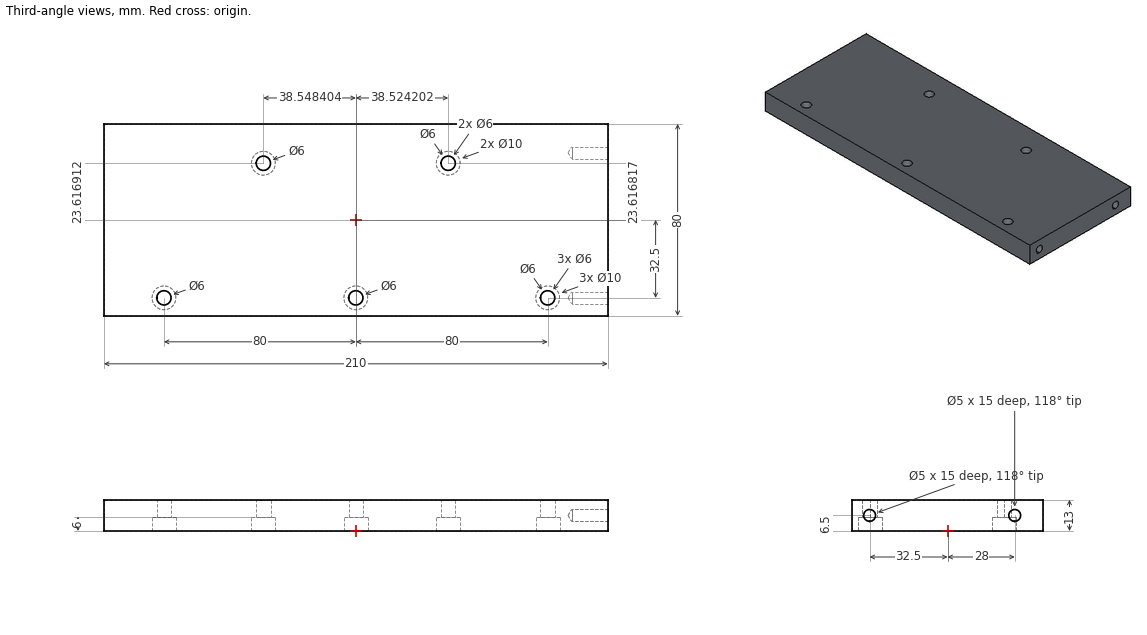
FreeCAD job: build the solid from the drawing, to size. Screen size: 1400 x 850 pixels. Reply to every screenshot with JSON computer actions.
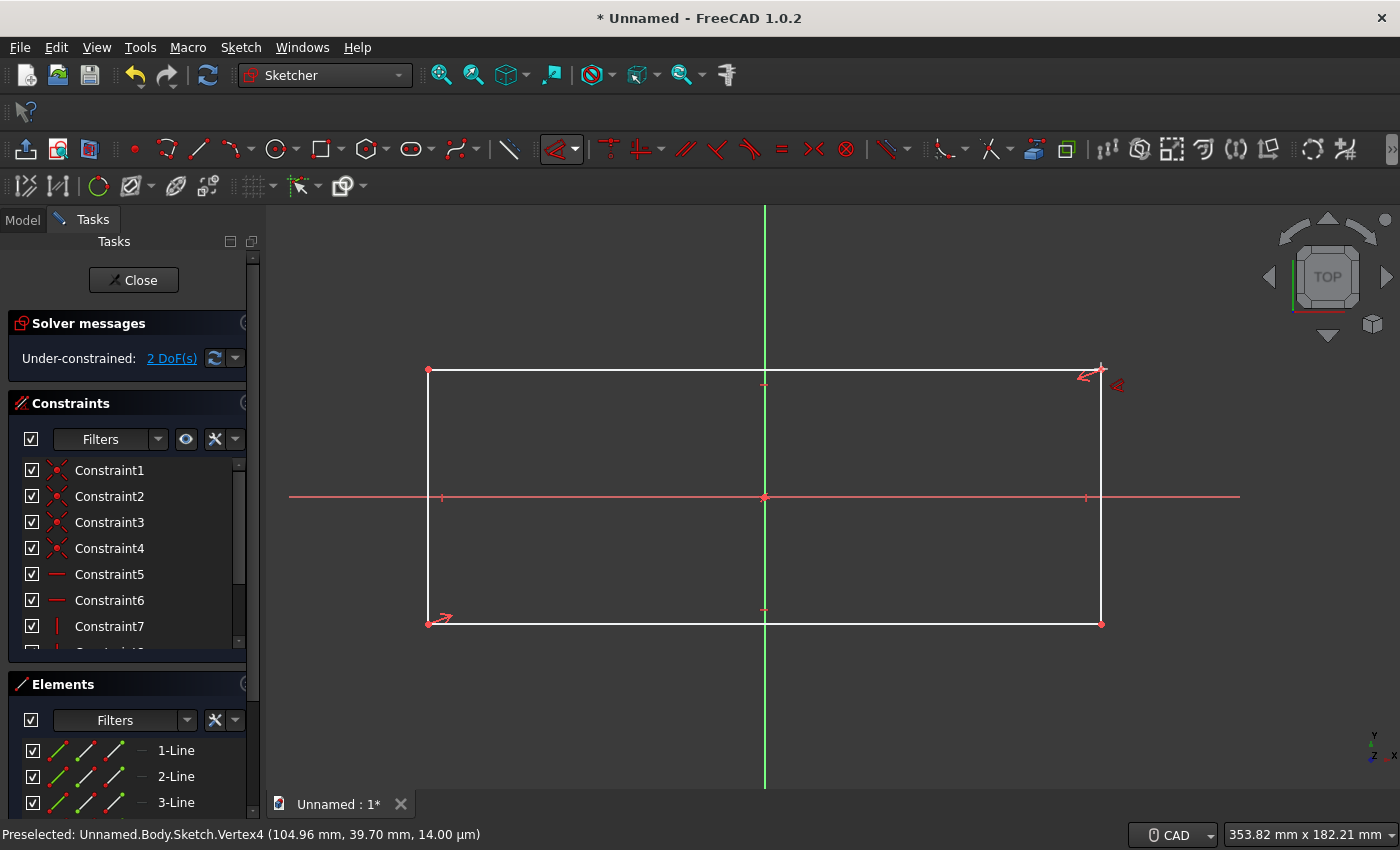
{"action": "left_click", "coordinate": [1101, 548]}
{"action": "left_click", "coordinate": [1135, 439]}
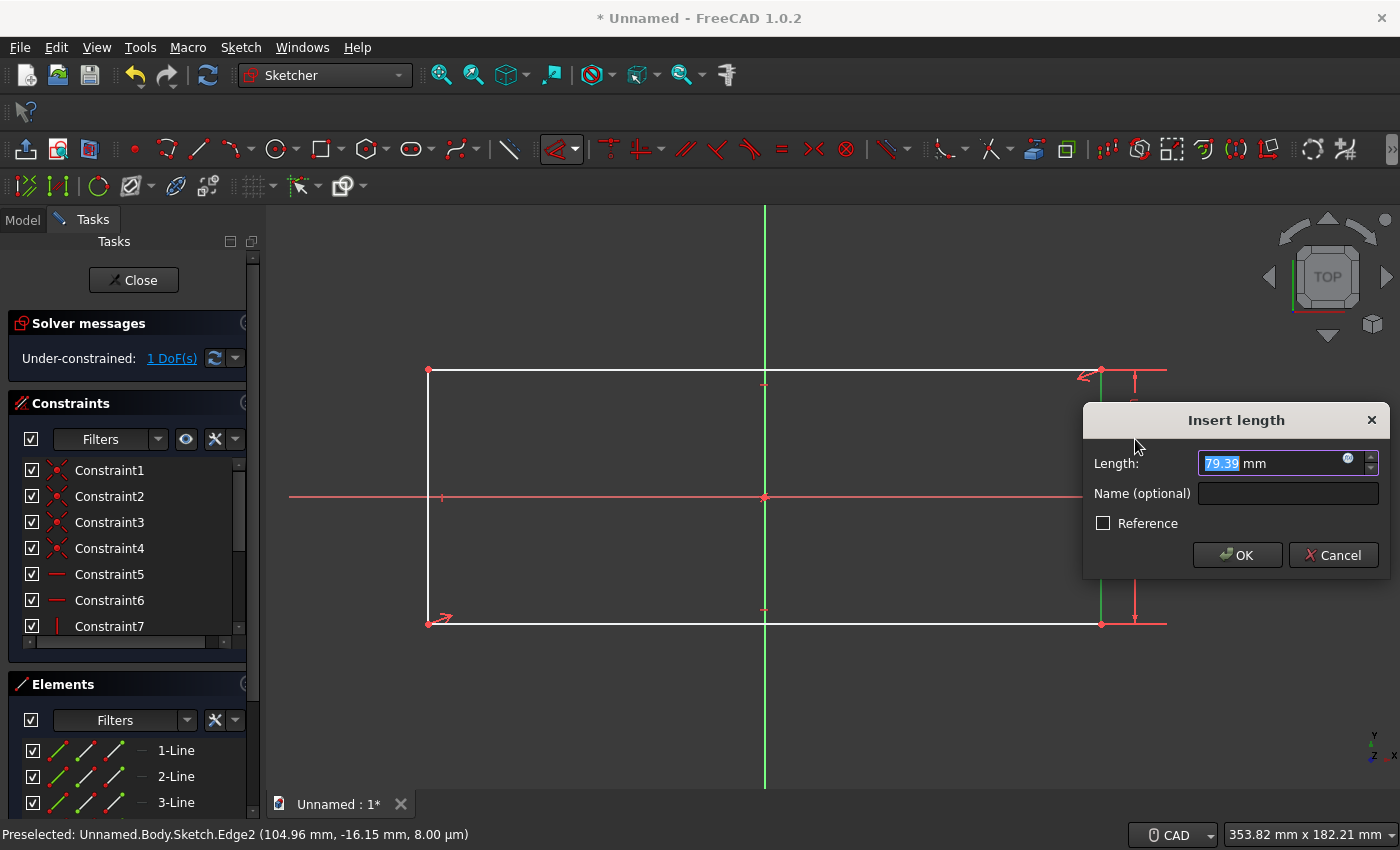
{"action": "type", "text": "80"}
{"action": "key", "text": "Return"}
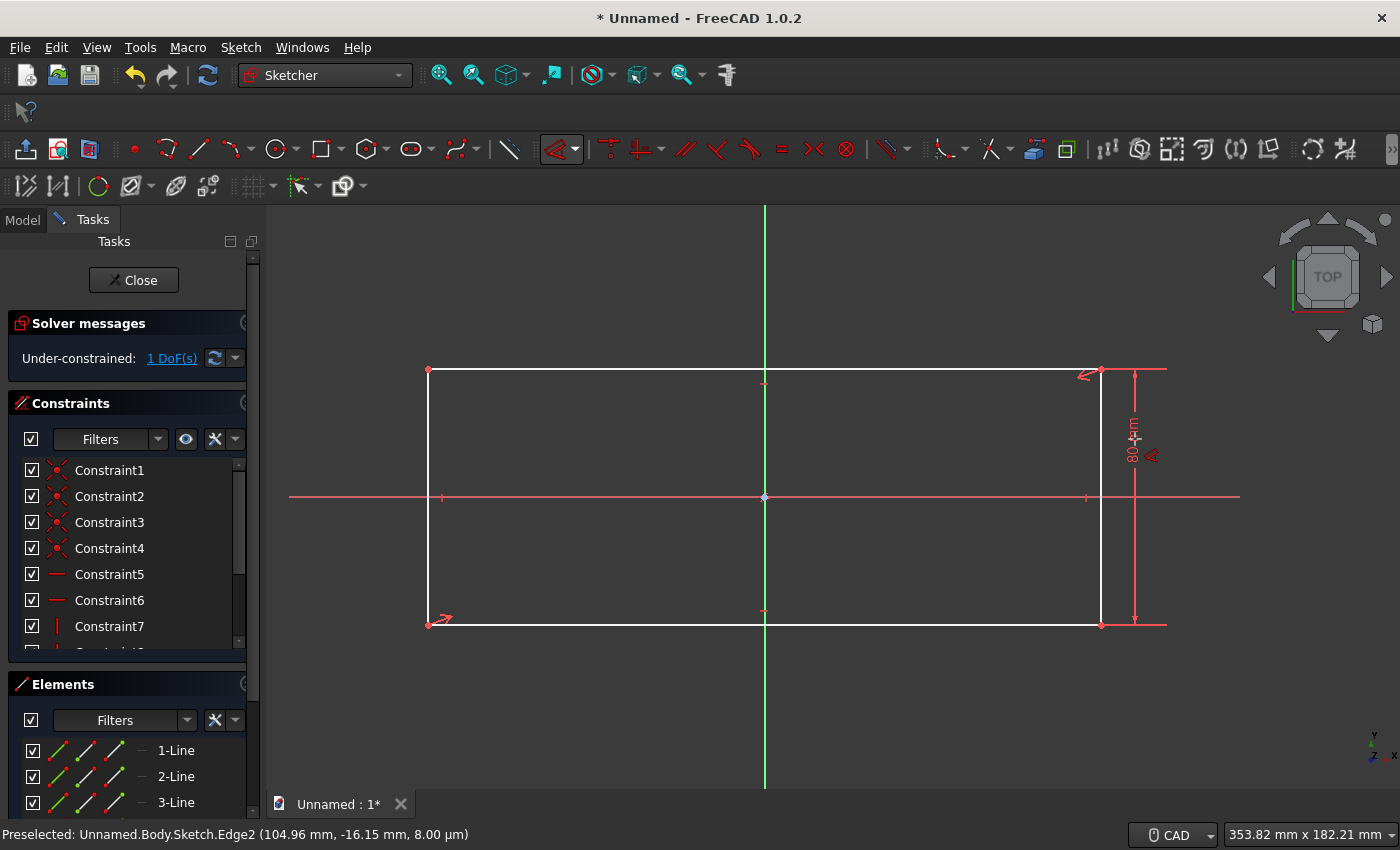
{"action": "left_click", "coordinate": [630, 625]}
{"action": "left_click", "coordinate": [610, 659]}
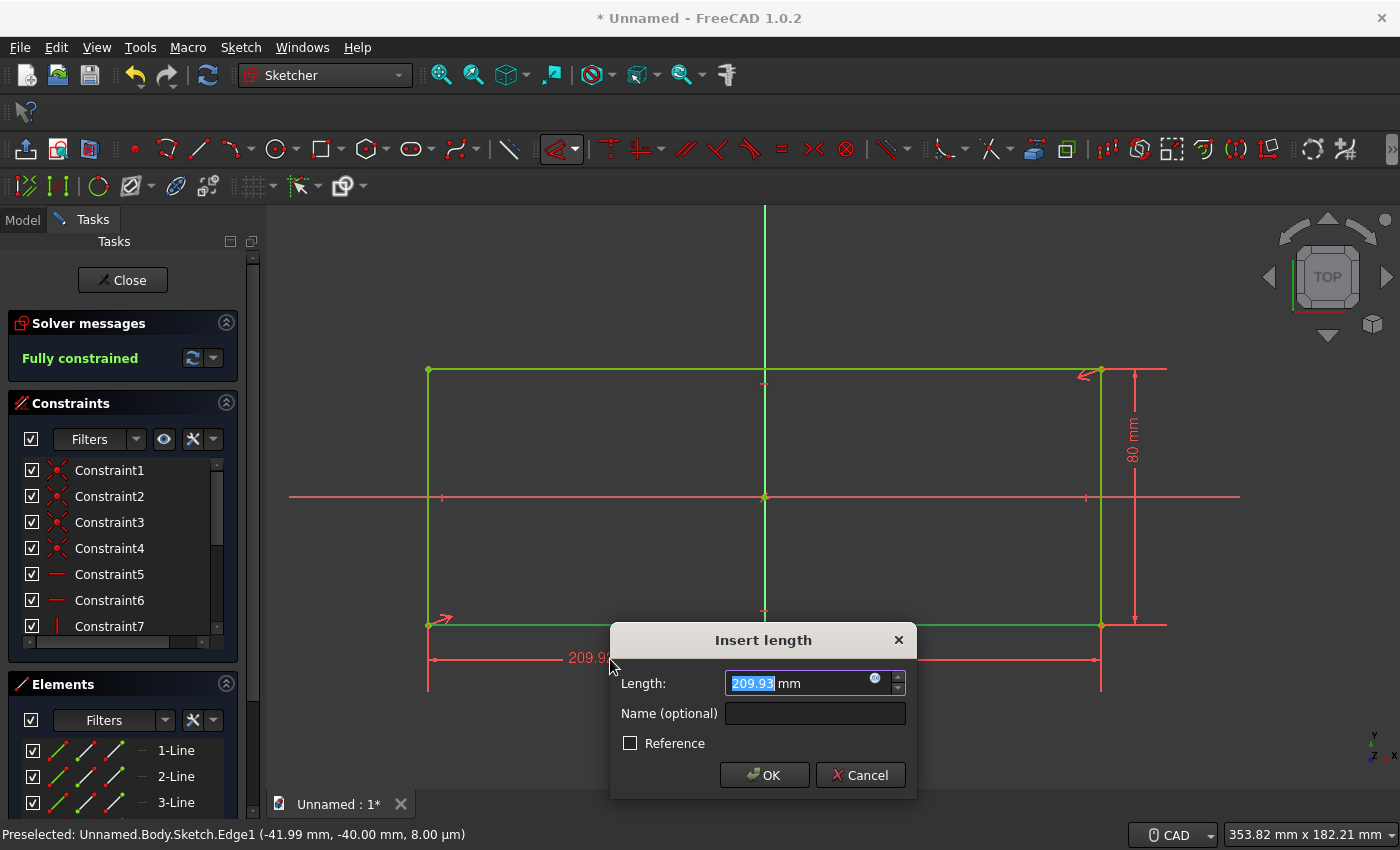
{"action": "type", "text": "210"}
{"action": "key", "text": "Return"}
{"action": "key", "text": "Escape"}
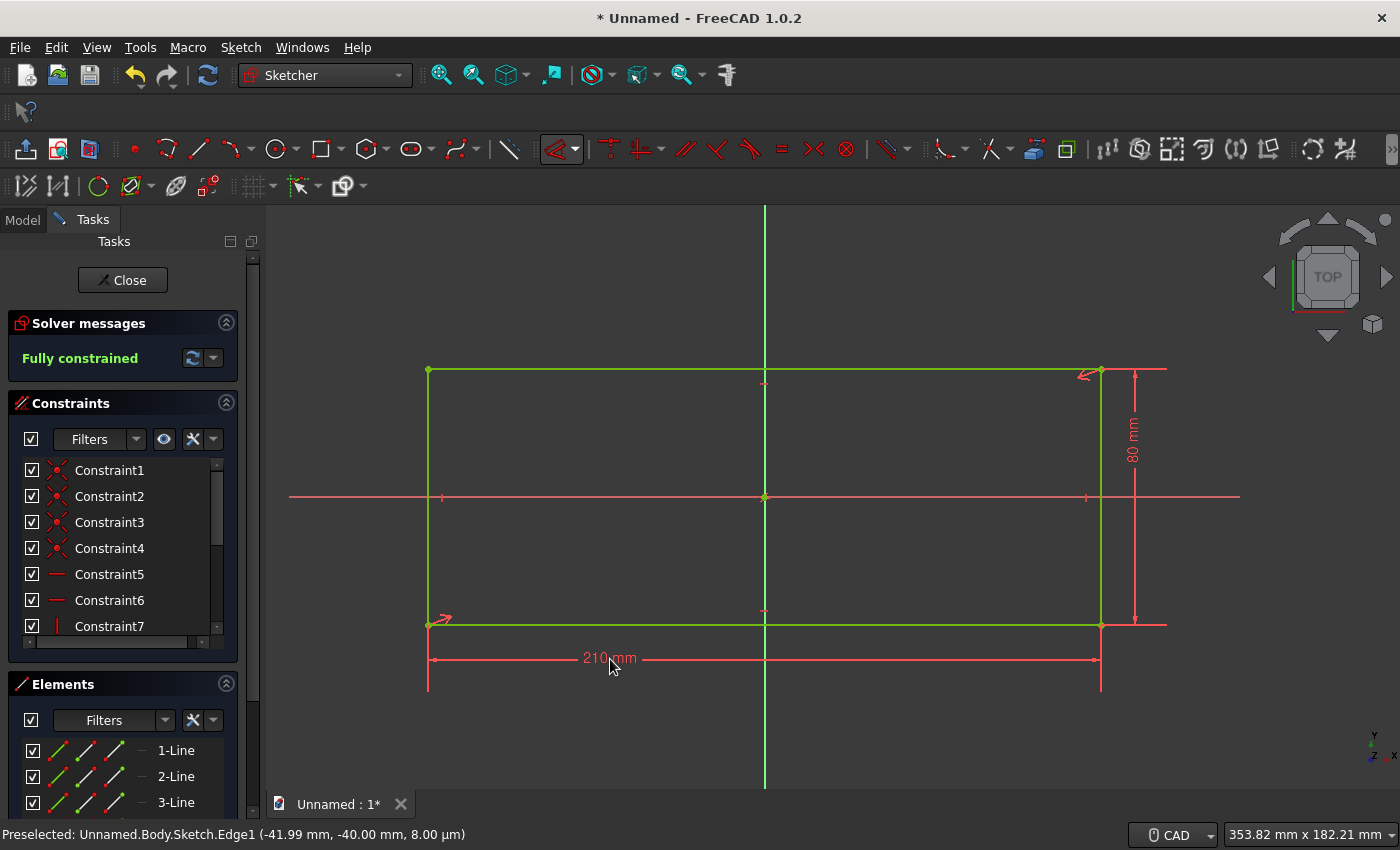
{"action": "left_click", "coordinate": [123, 280]}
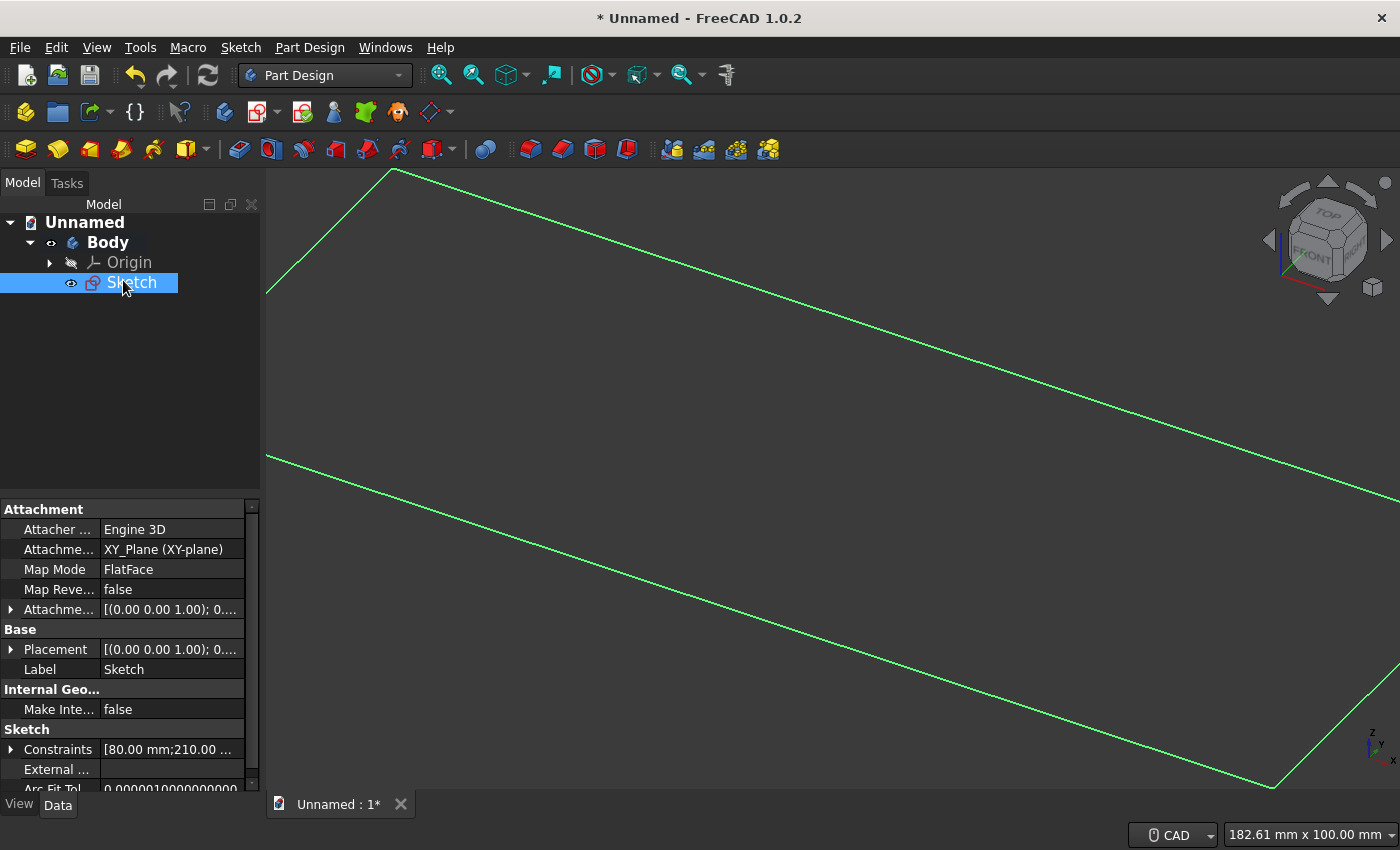
{"action": "left_click", "coordinate": [26, 150]}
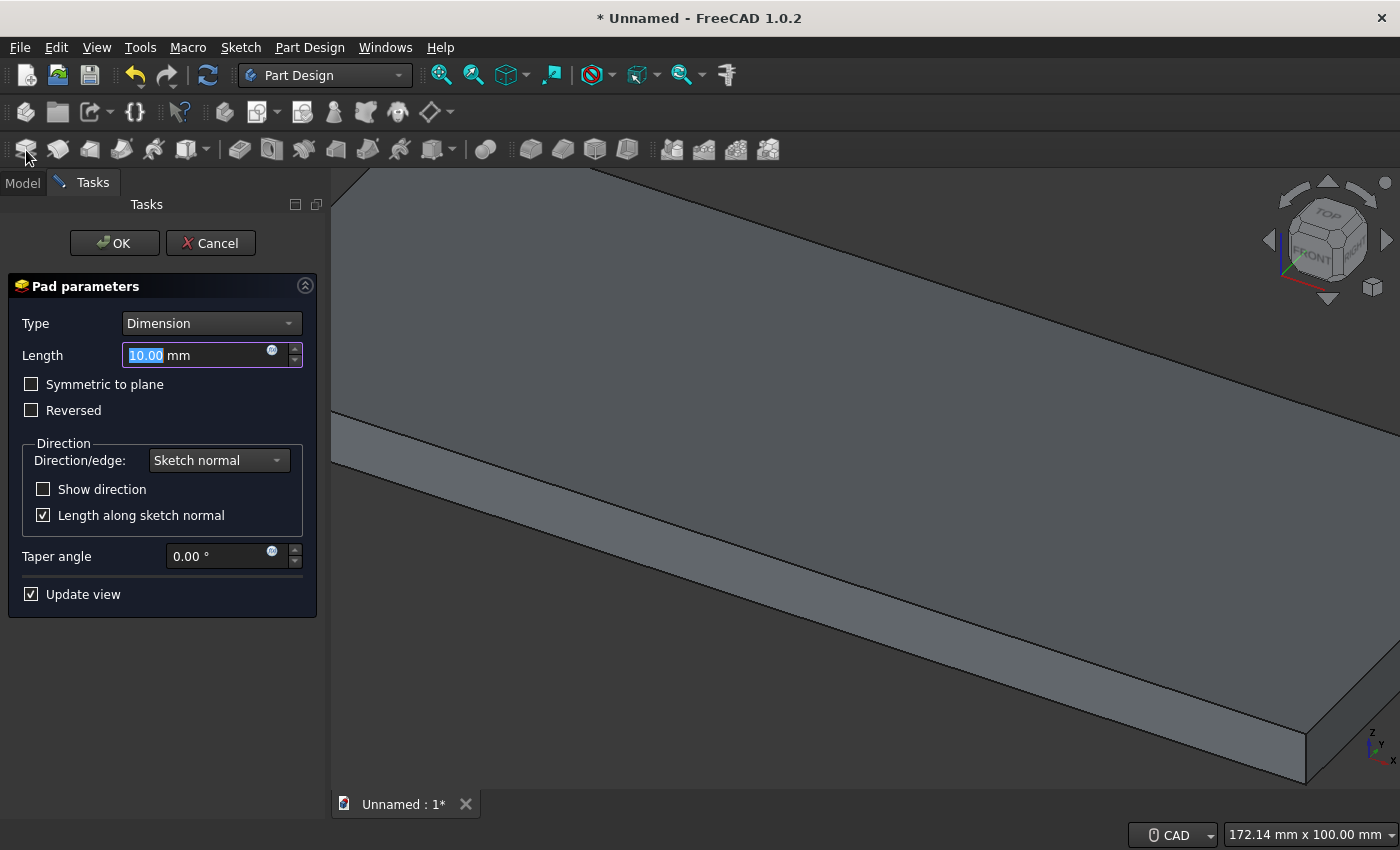
{"action": "type", "text": "13"}
{"action": "key", "text": "Tab"}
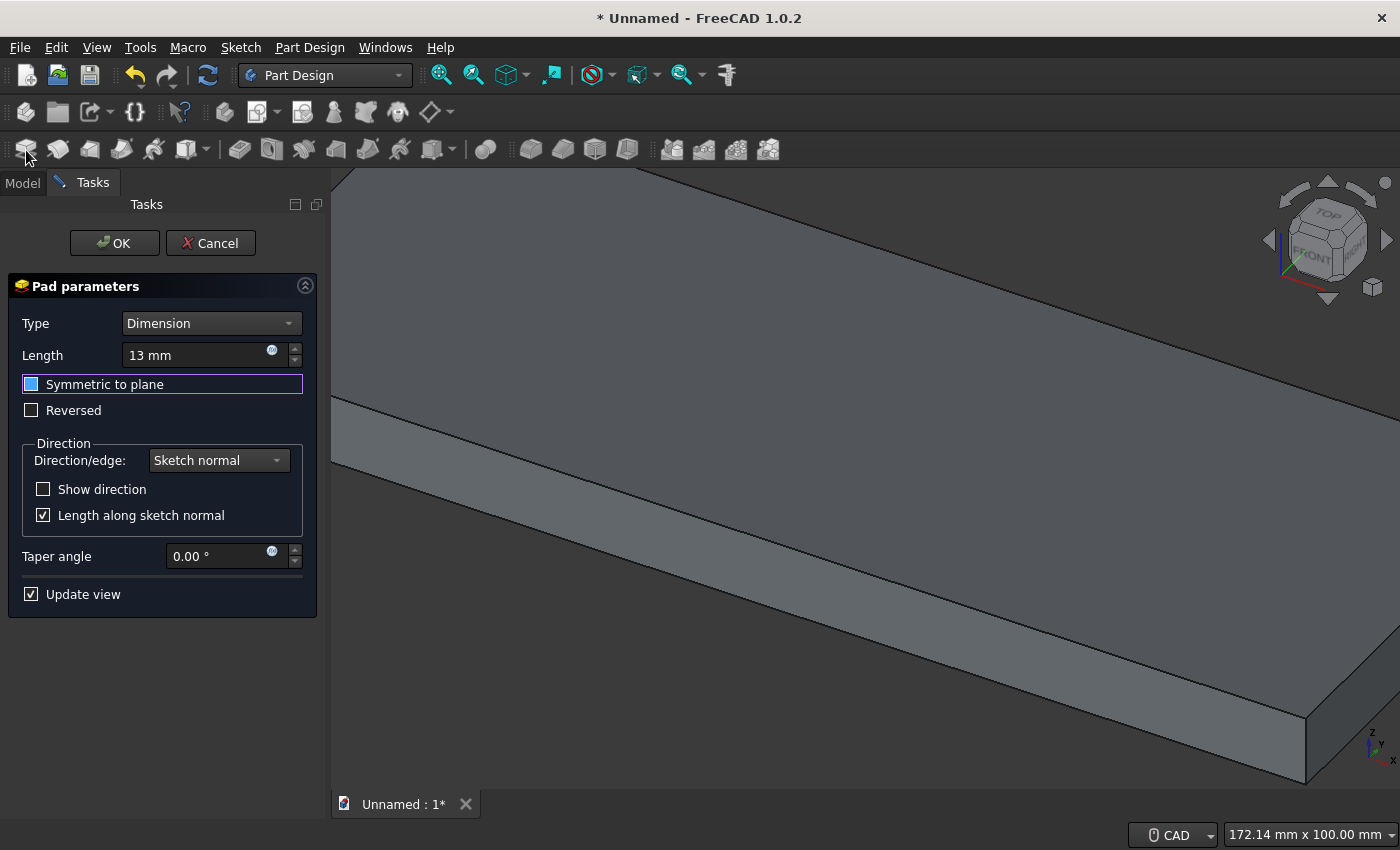
{"action": "left_click", "coordinate": [115, 243]}